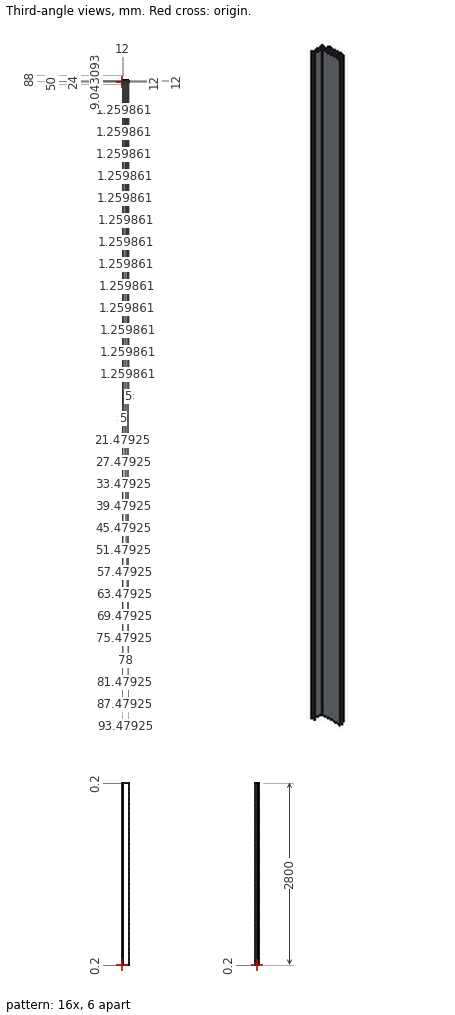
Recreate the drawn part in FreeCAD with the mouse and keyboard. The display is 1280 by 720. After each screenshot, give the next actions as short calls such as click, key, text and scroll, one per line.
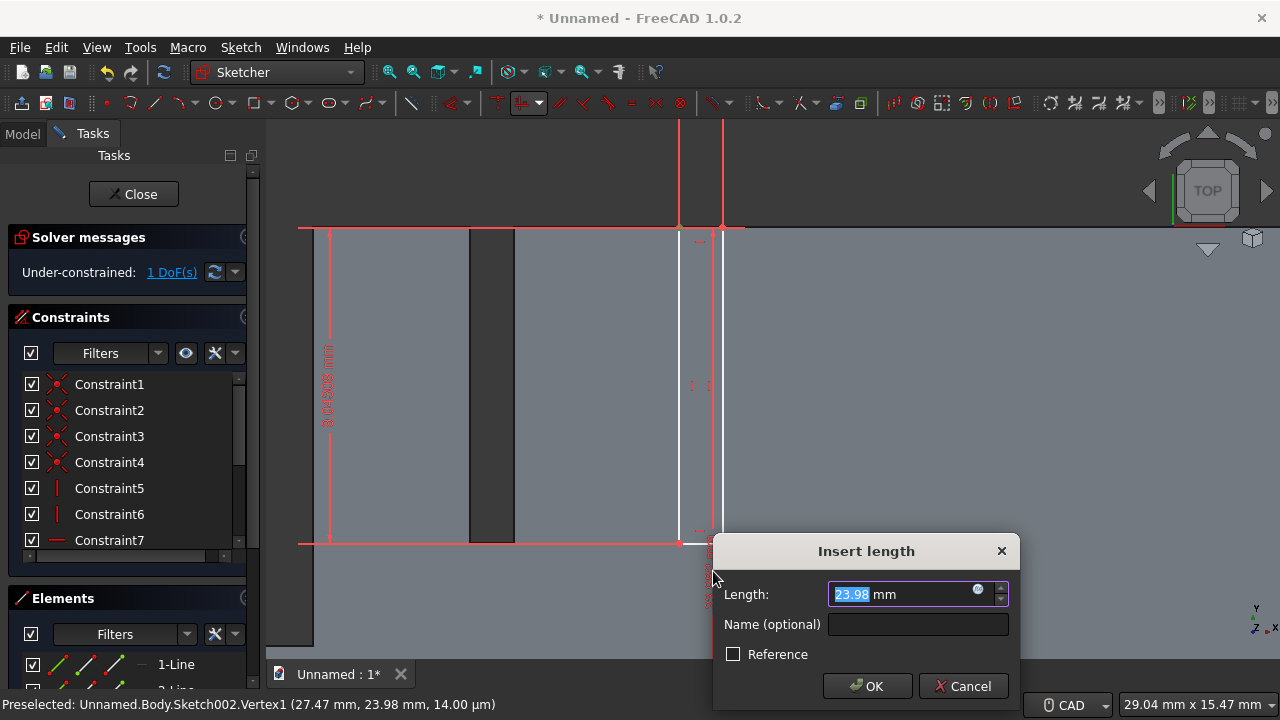
text(24)
key(Return)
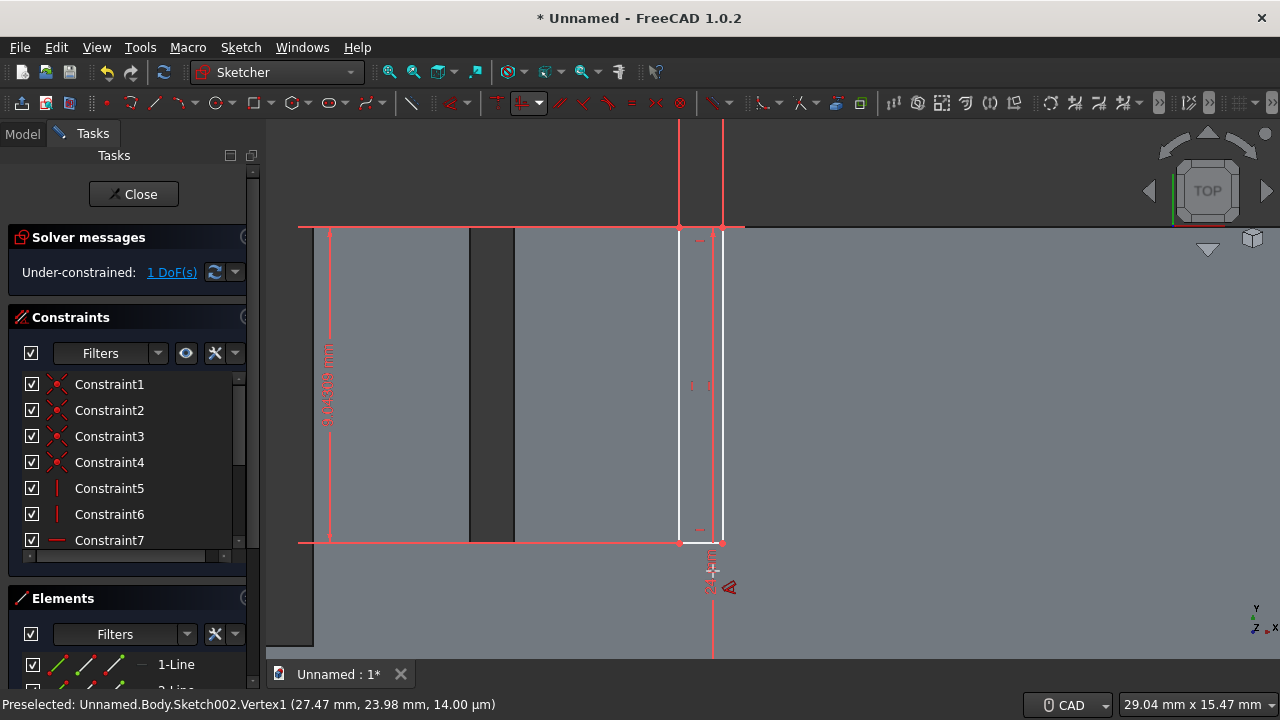
click(679, 227)
click(486, 193)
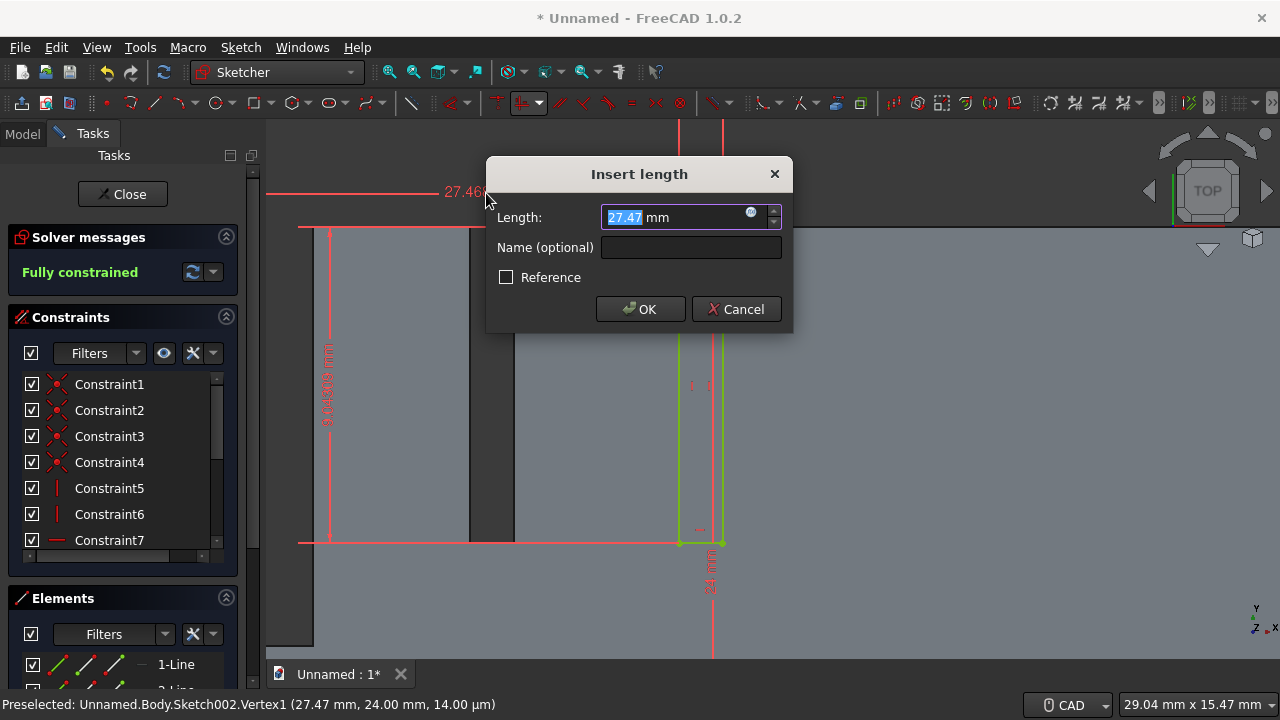
text(27.47925)
key(Return)
key(Escape)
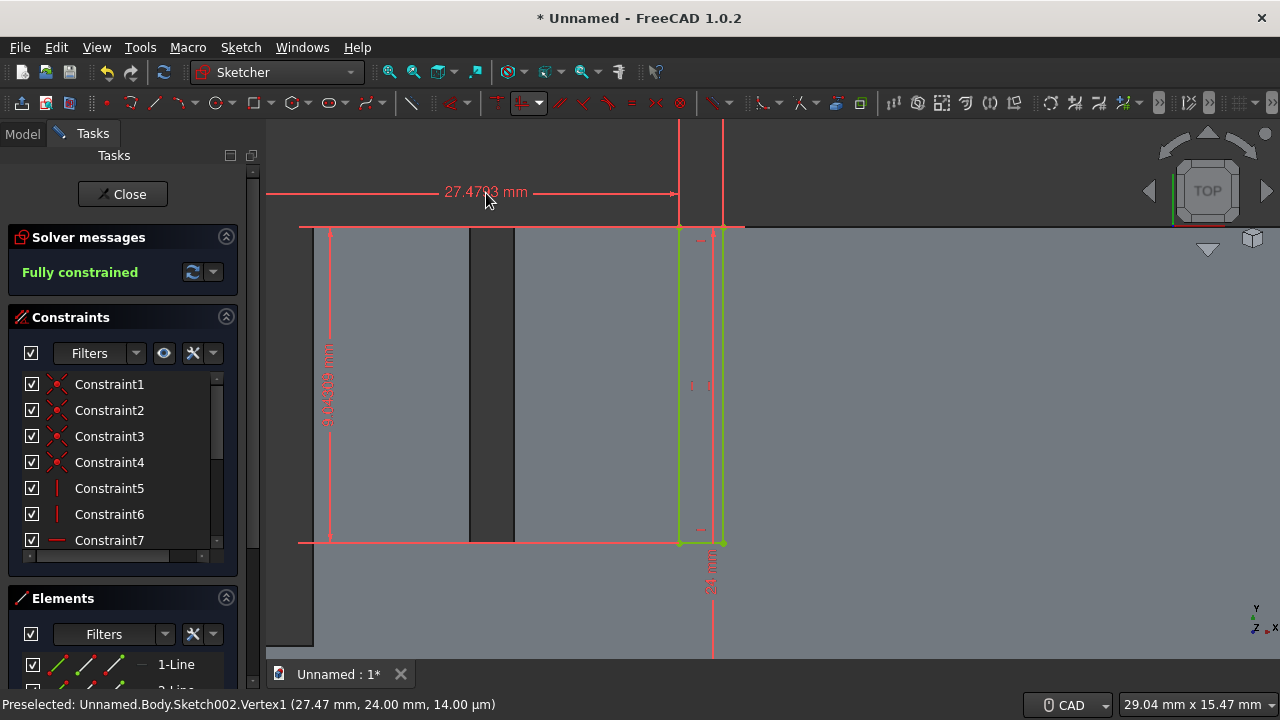
click(123, 194)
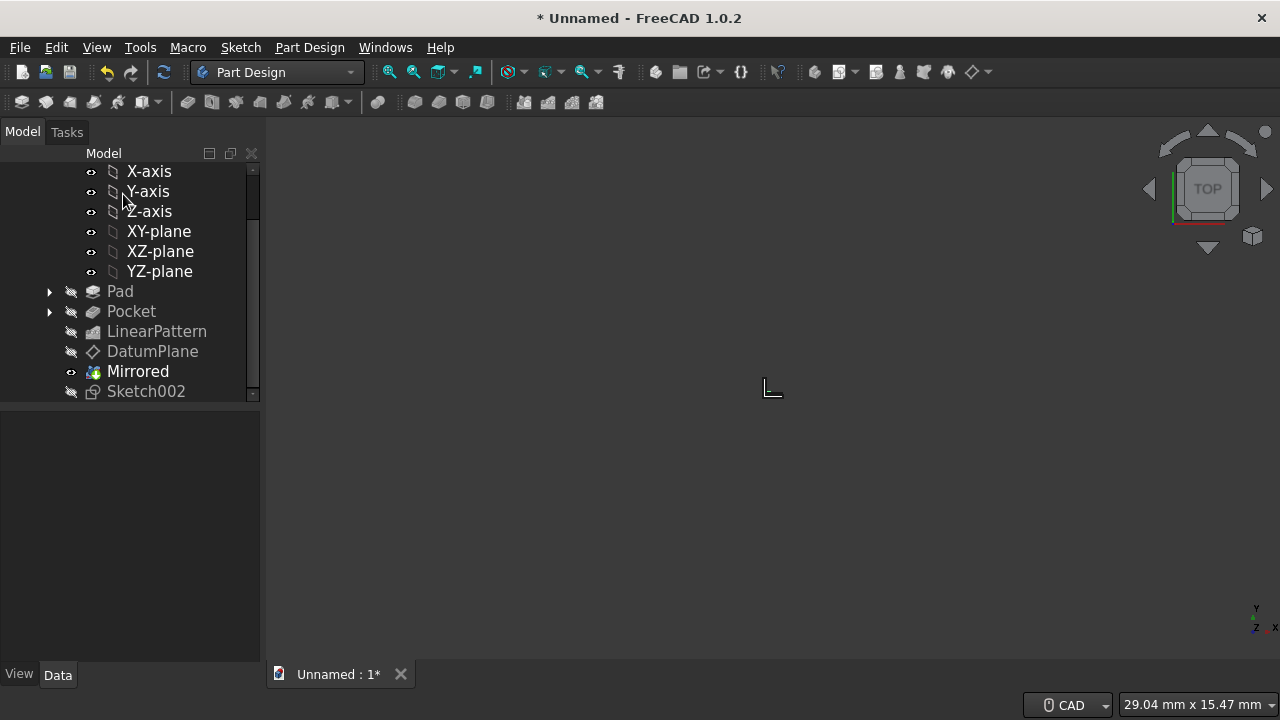
click(188, 102)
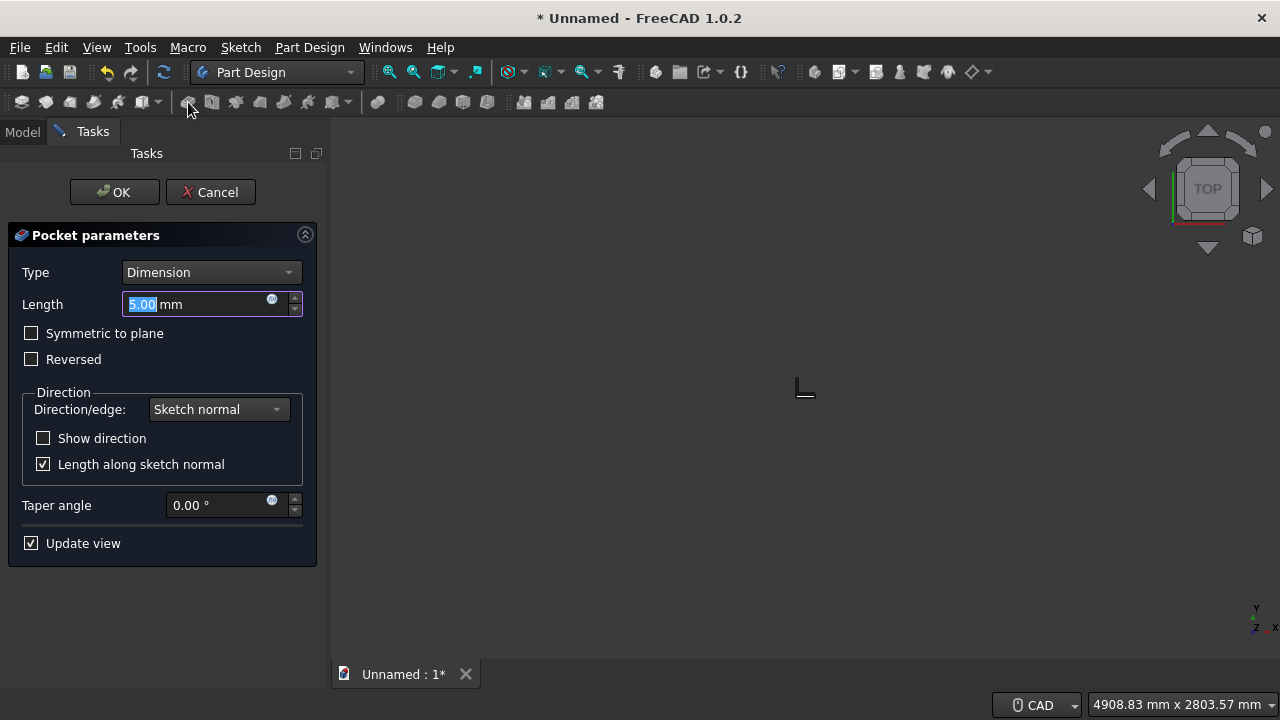
text(0.2)
key(Tab)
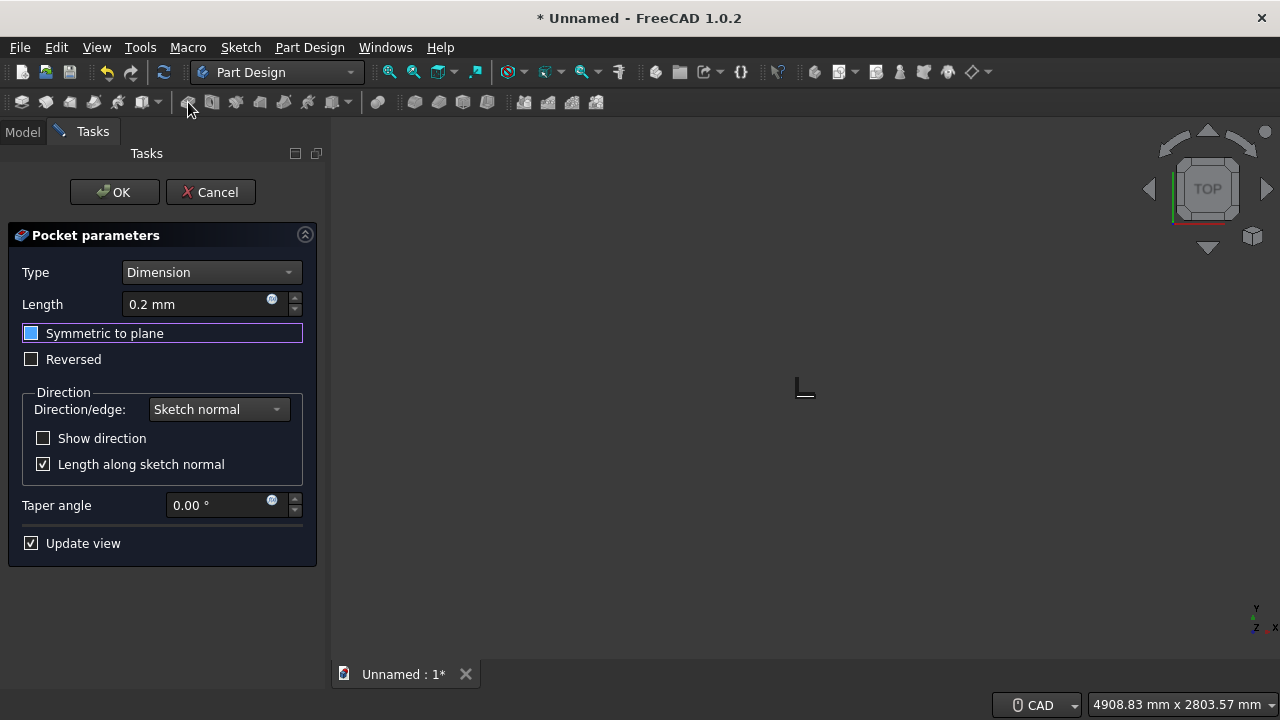
click(30, 359)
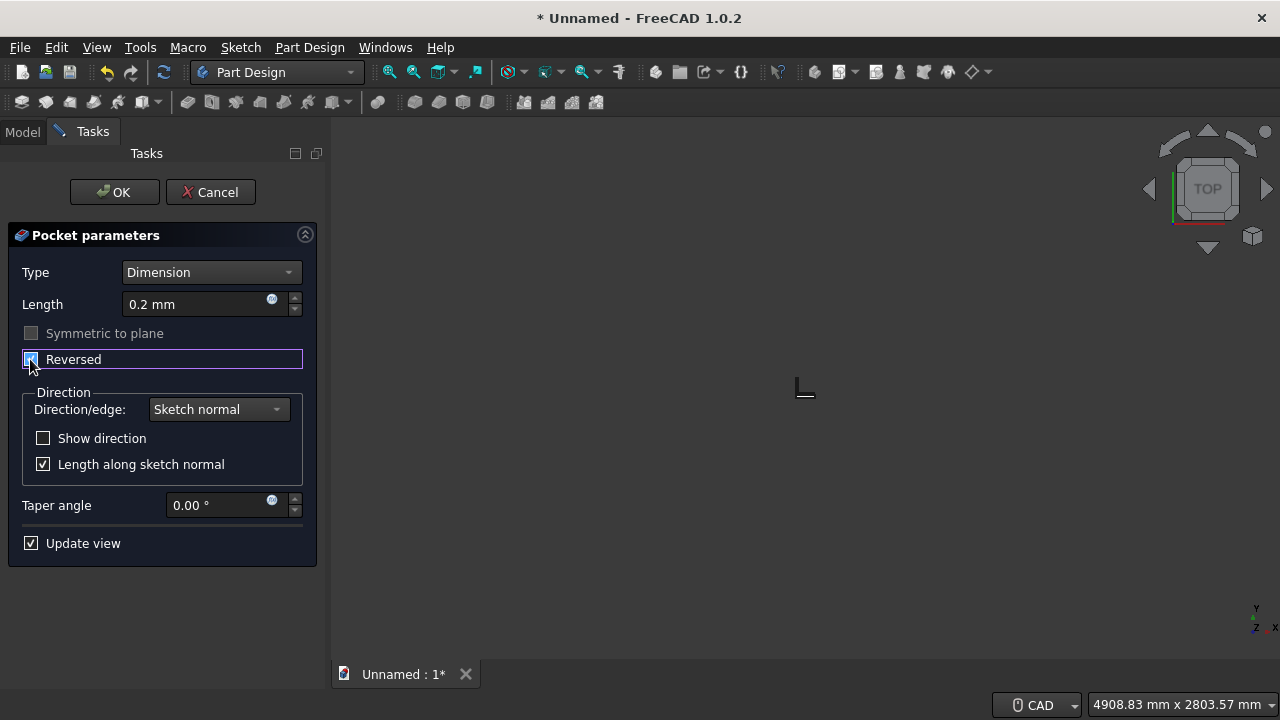
click(115, 192)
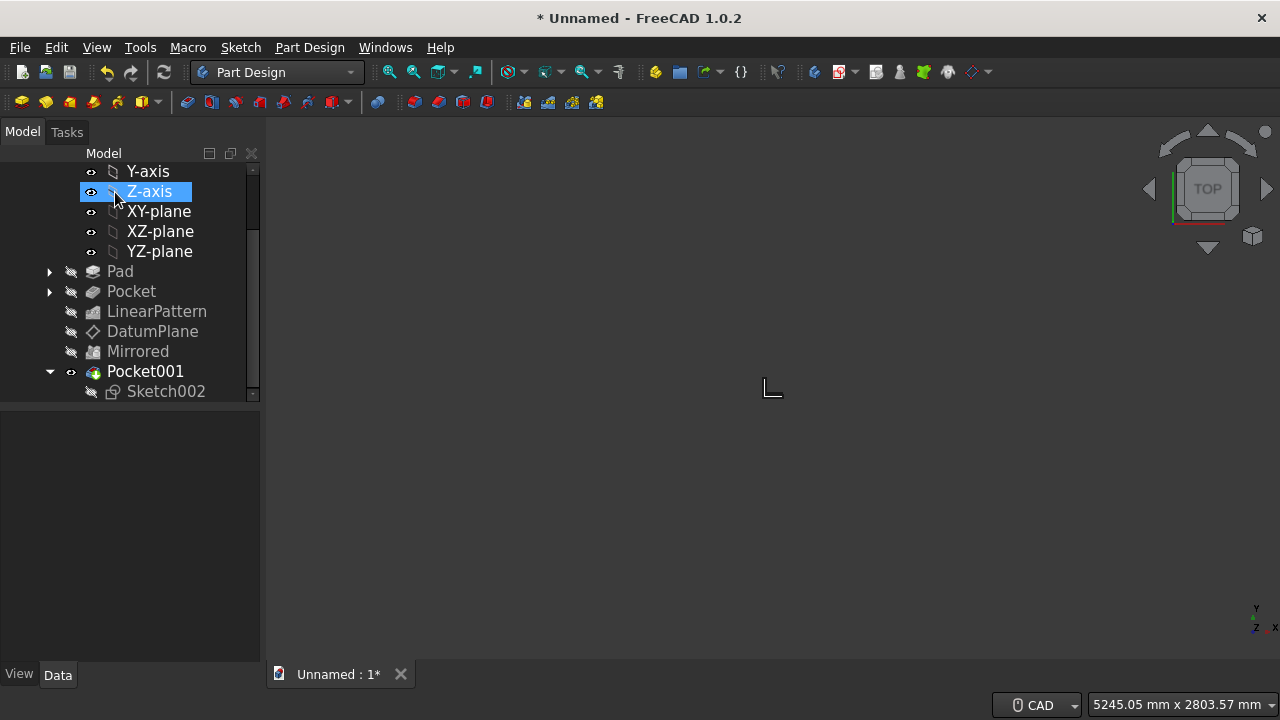
click(390, 72)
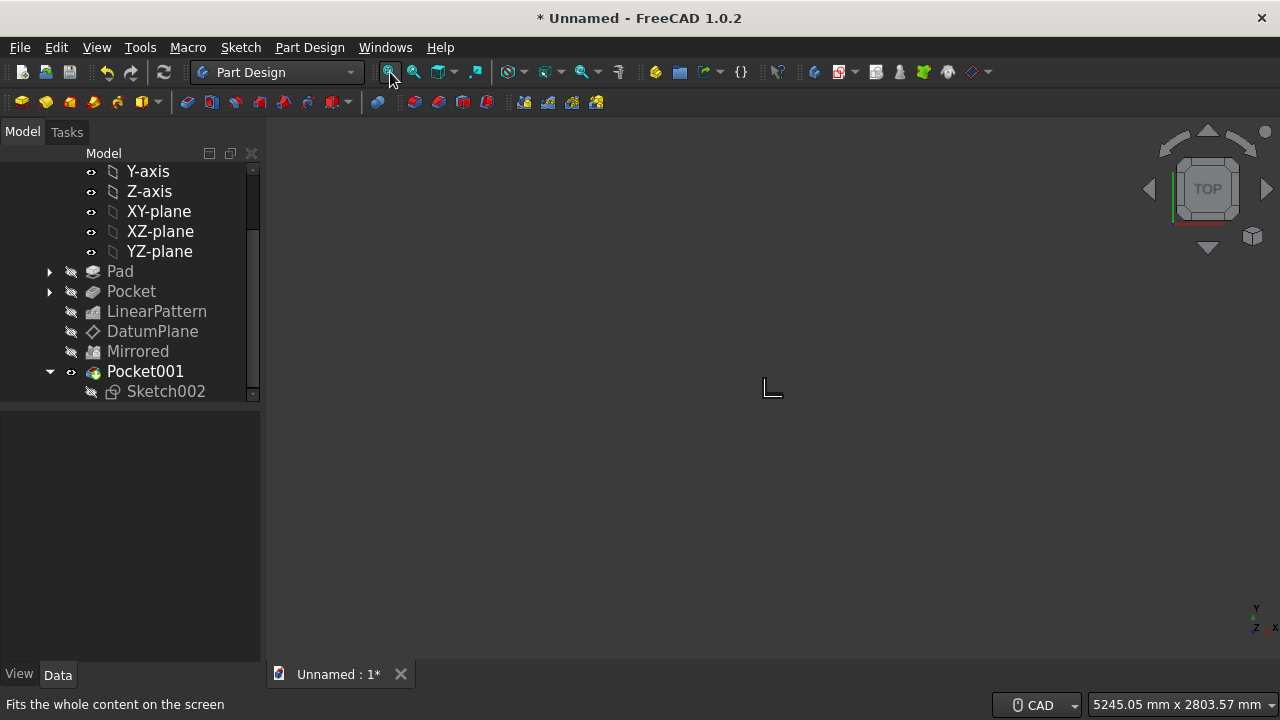
click(840, 72)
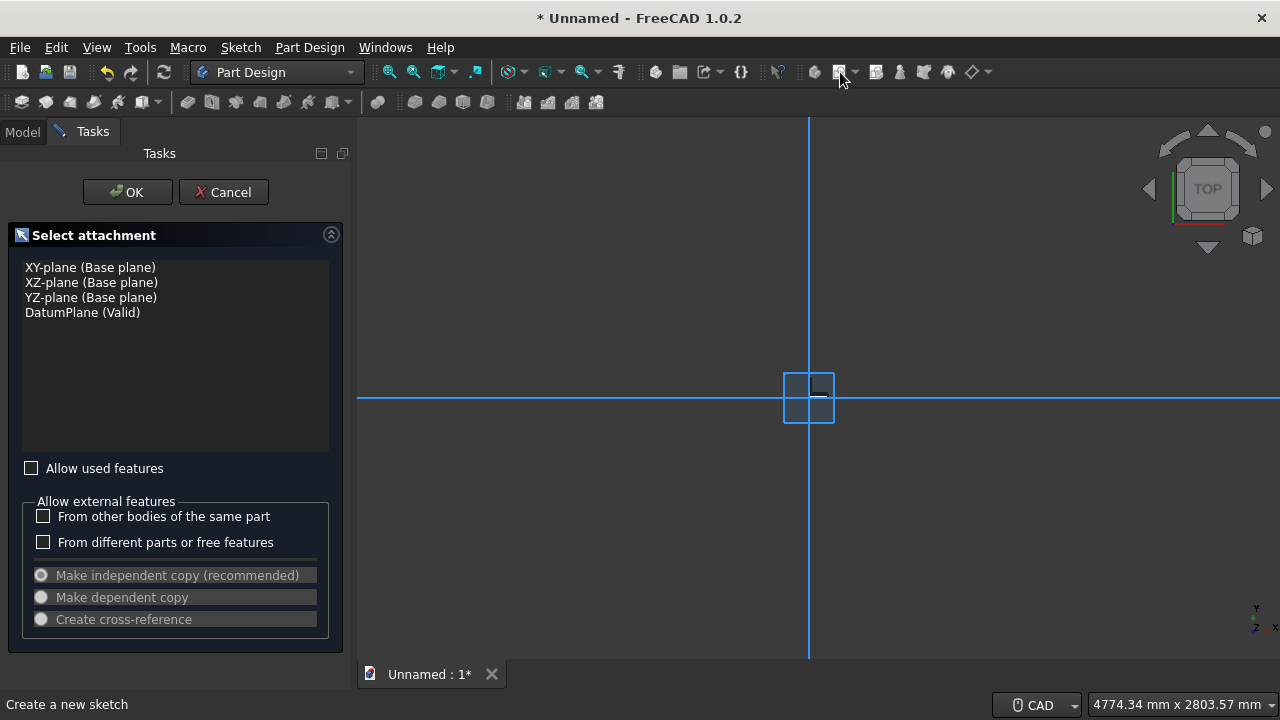
click(82, 268)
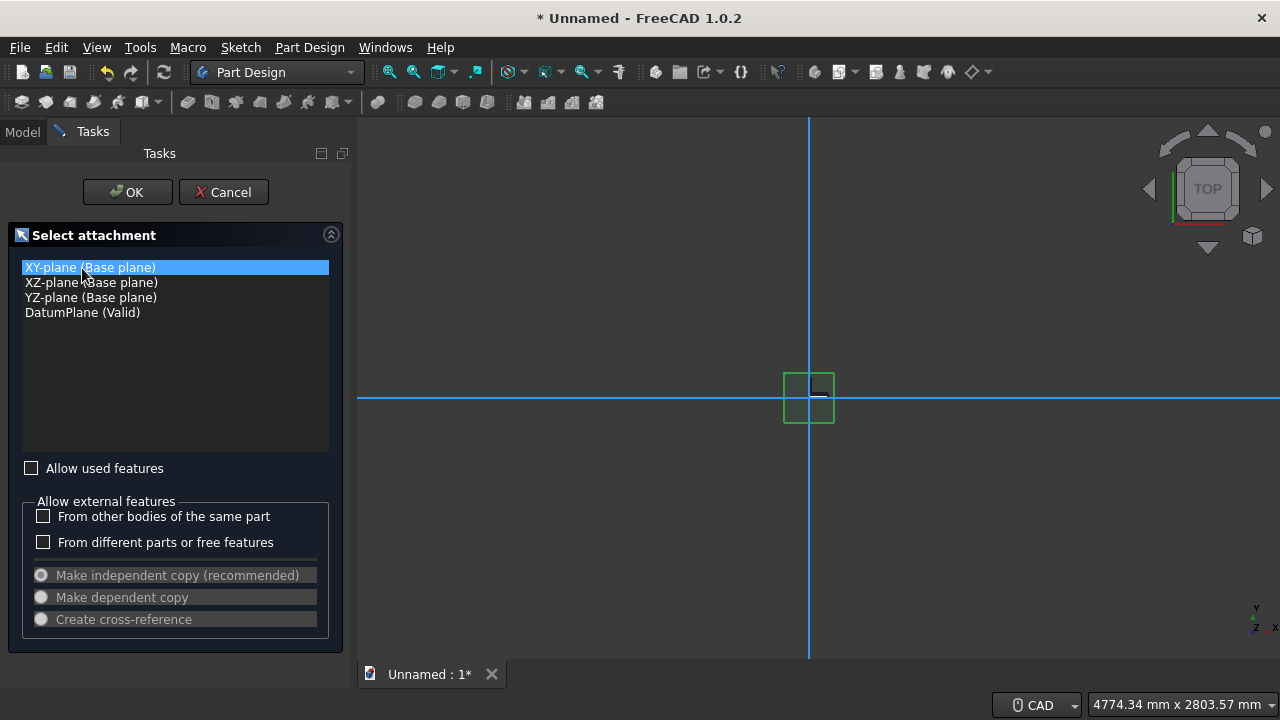
click(128, 192)